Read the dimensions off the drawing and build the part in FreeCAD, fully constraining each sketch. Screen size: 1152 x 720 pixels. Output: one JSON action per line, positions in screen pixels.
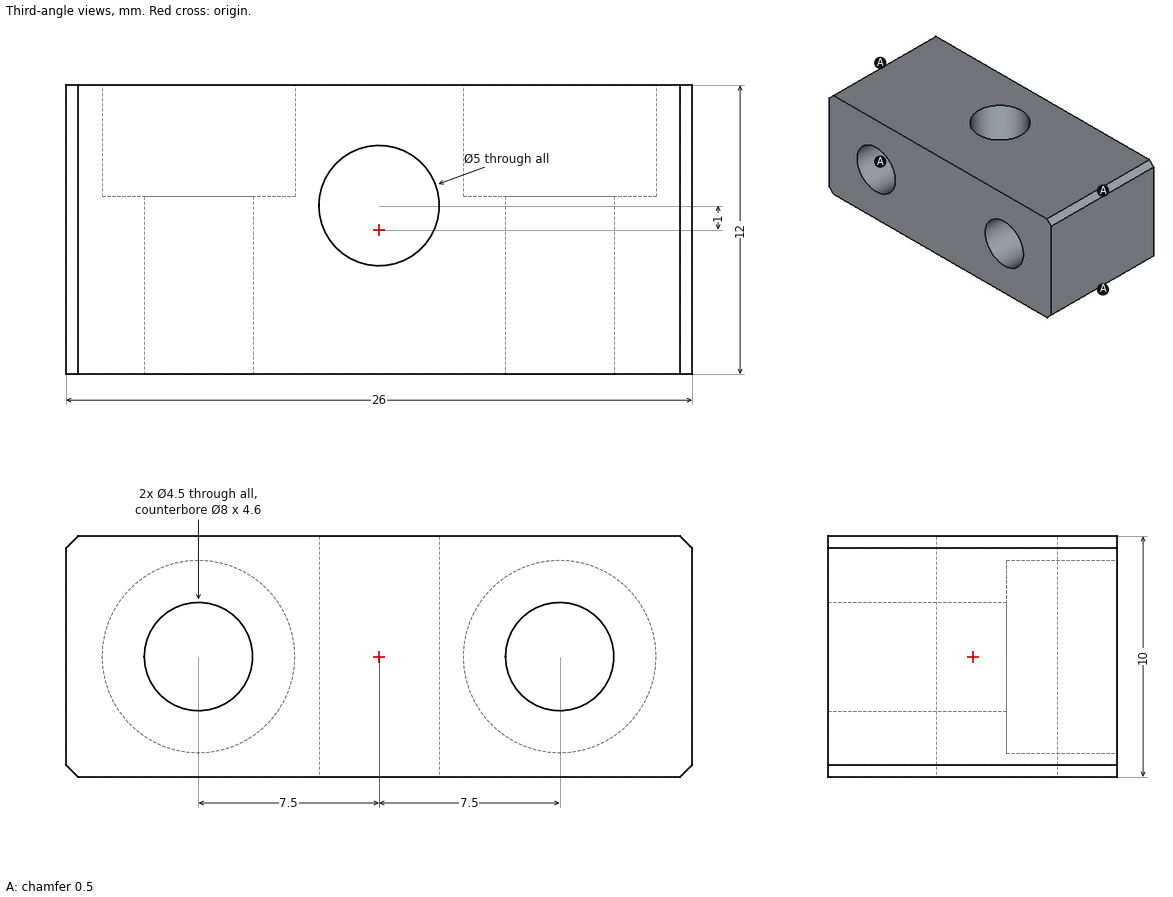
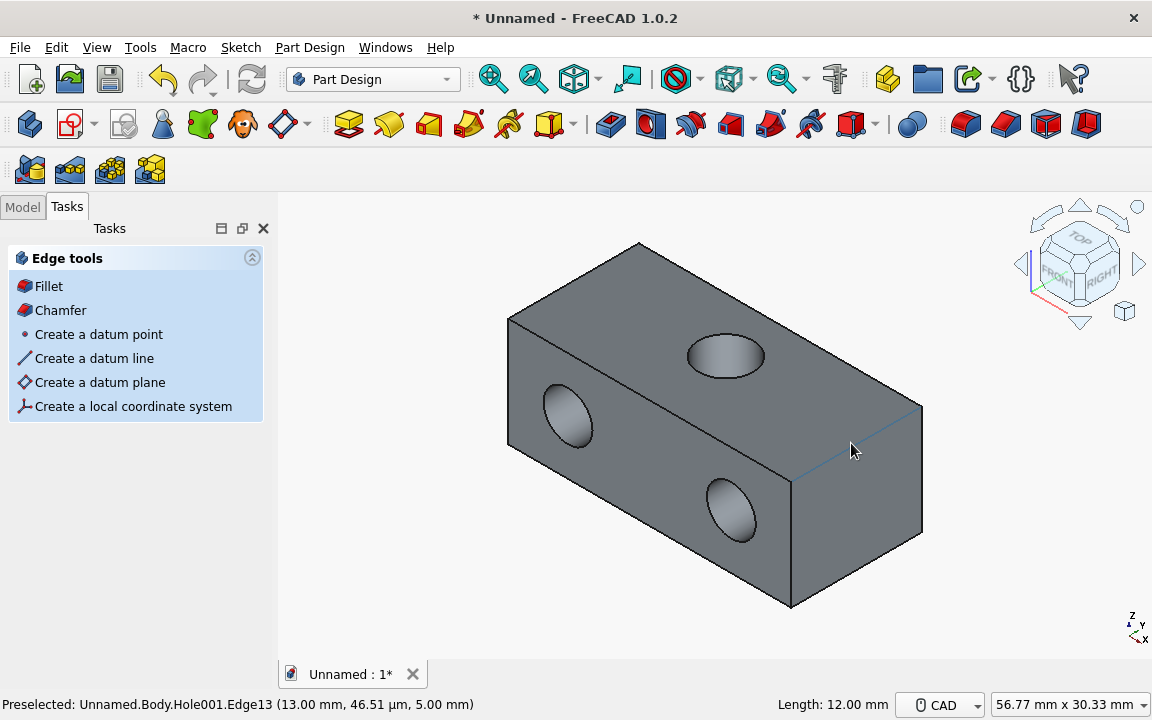
{"action": "key", "text": "2"}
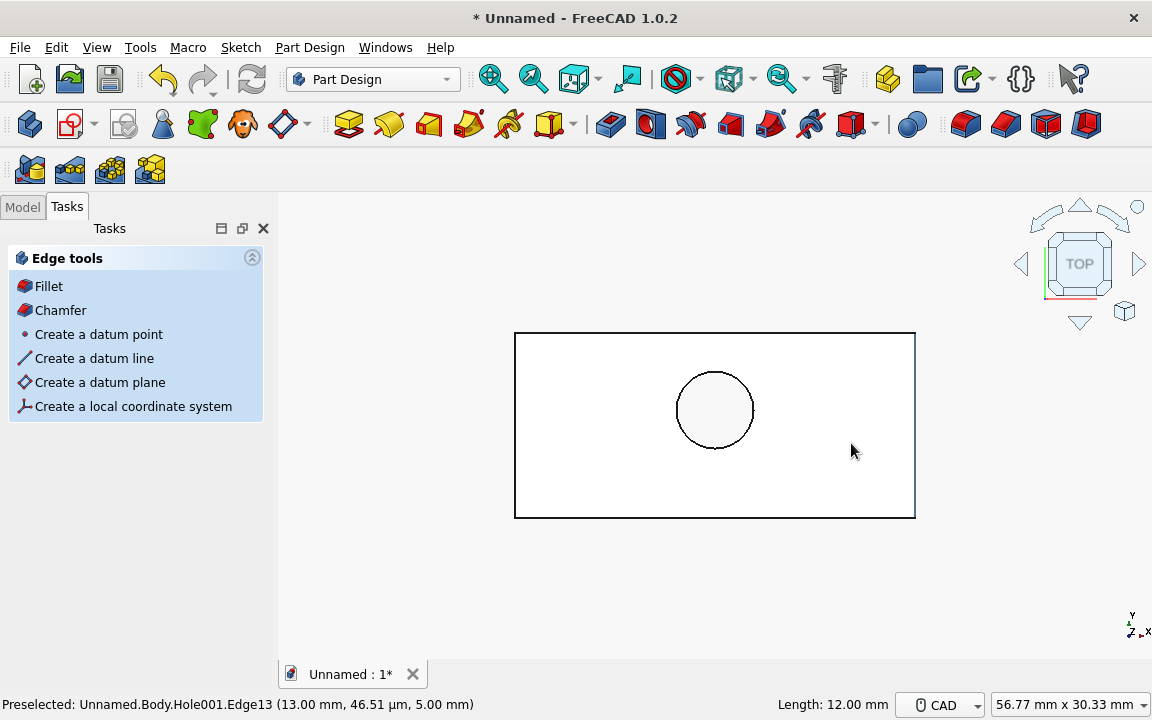
{"action": "left_click", "coordinate": [515, 424], "text": "ctrl"}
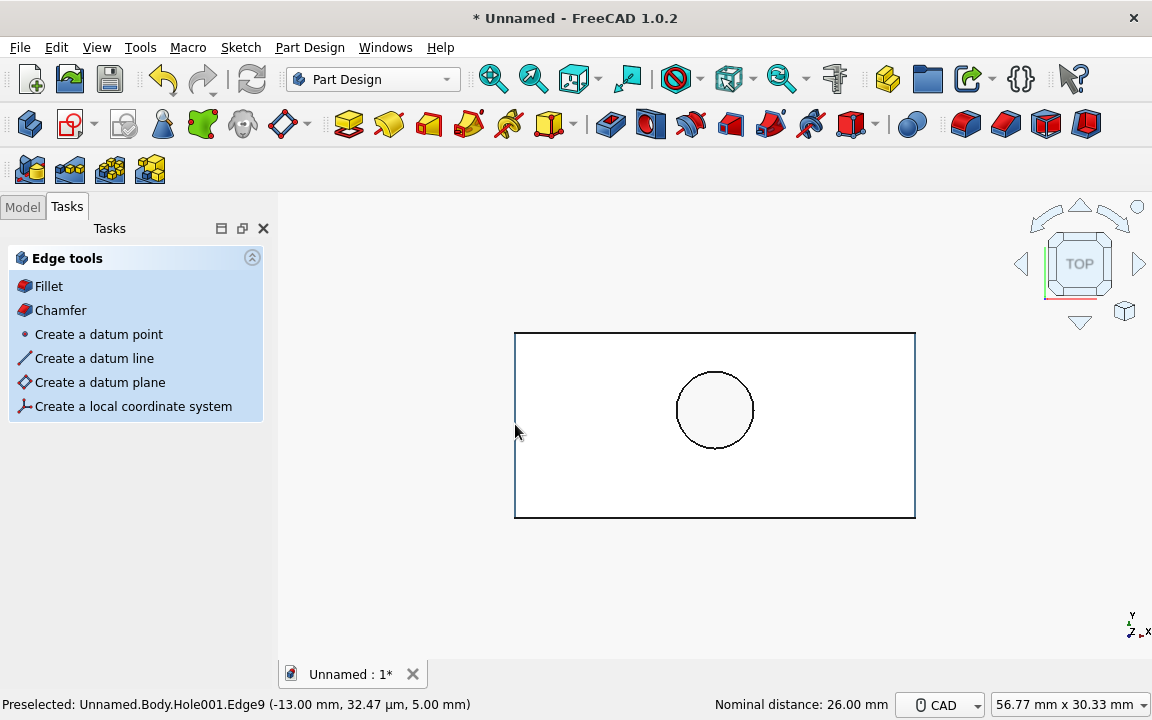
{"action": "key", "text": "0"}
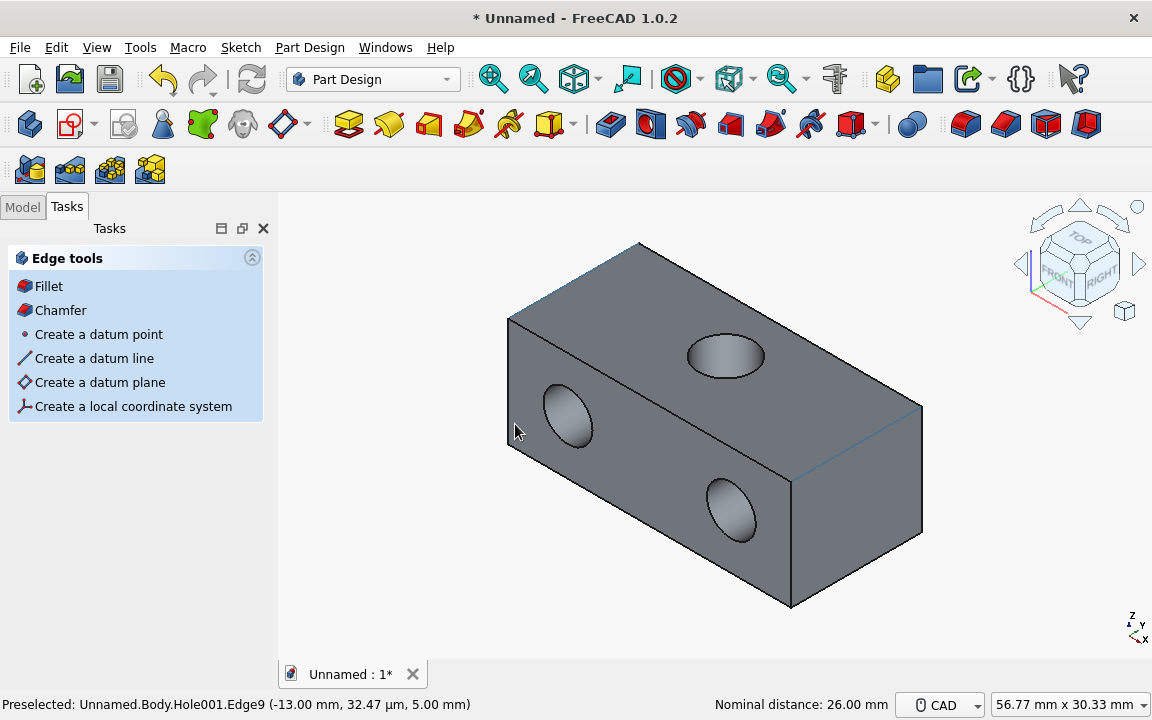
{"action": "key", "text": "1"}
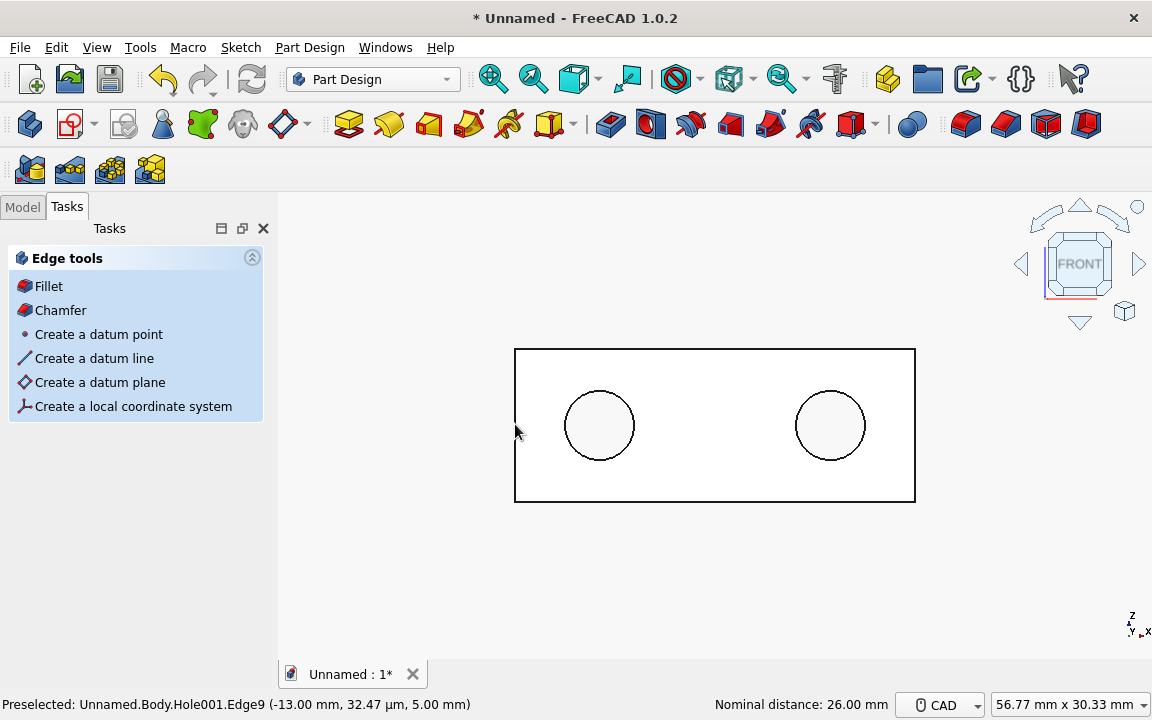
{"action": "key", "text": "3"}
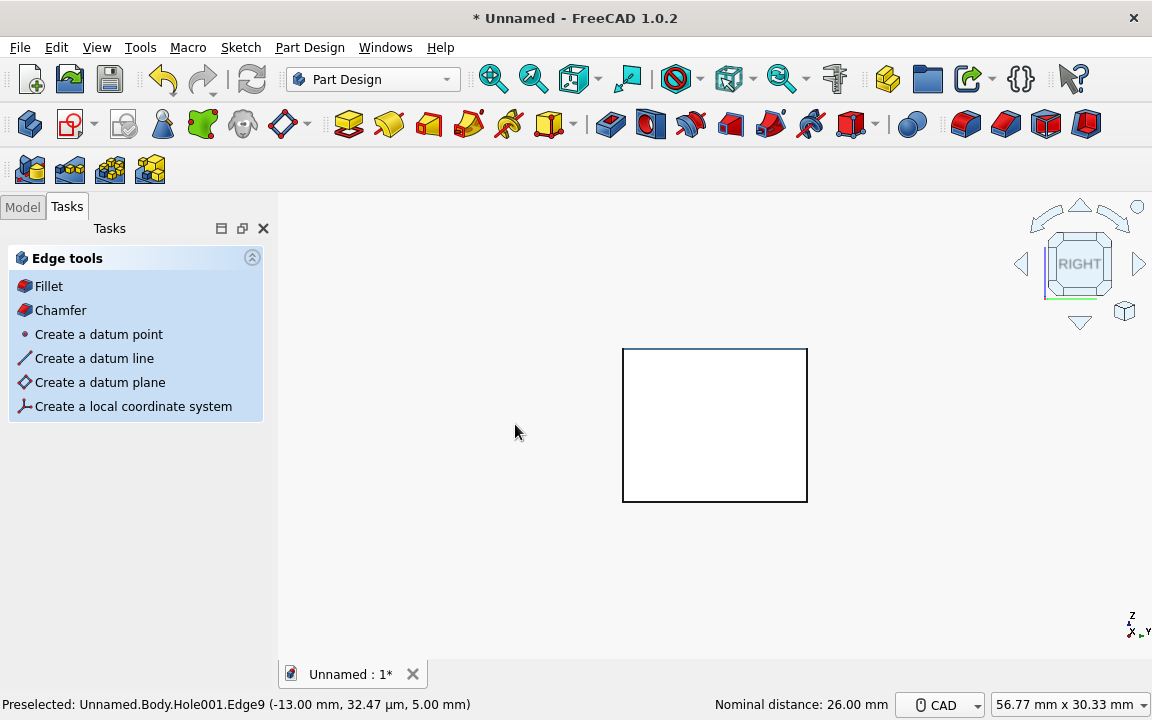
{"action": "key", "text": "v f"}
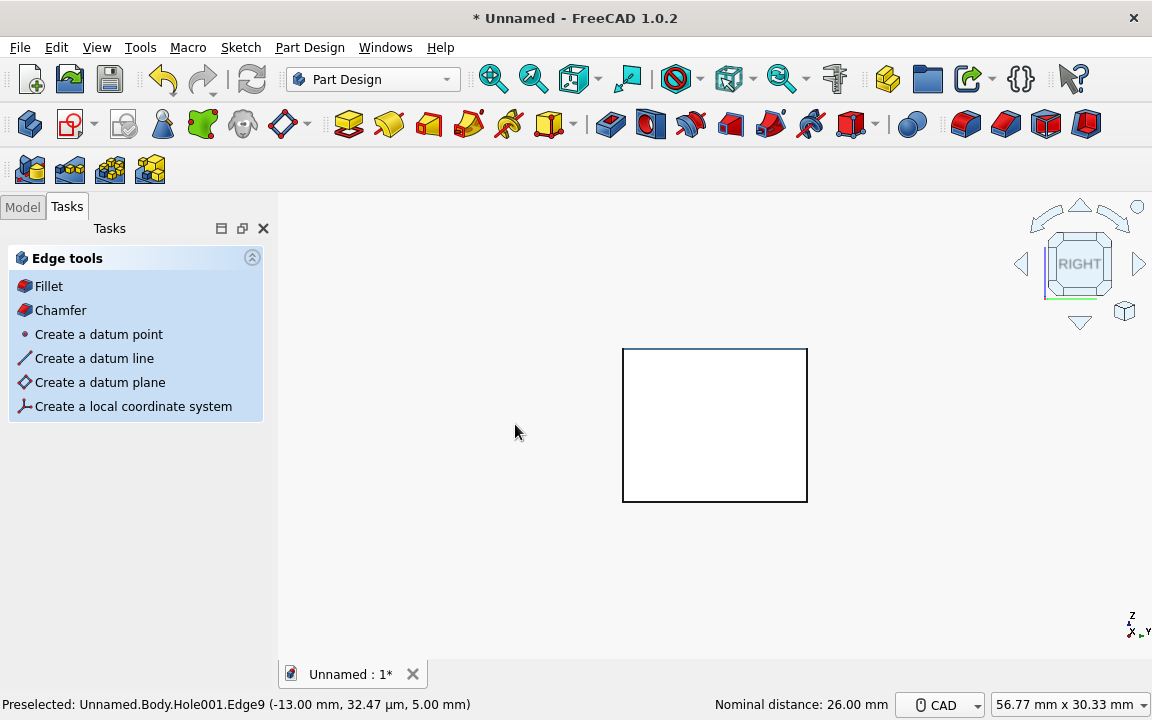
{"action": "left_click", "coordinate": [715, 501], "text": "ctrl"}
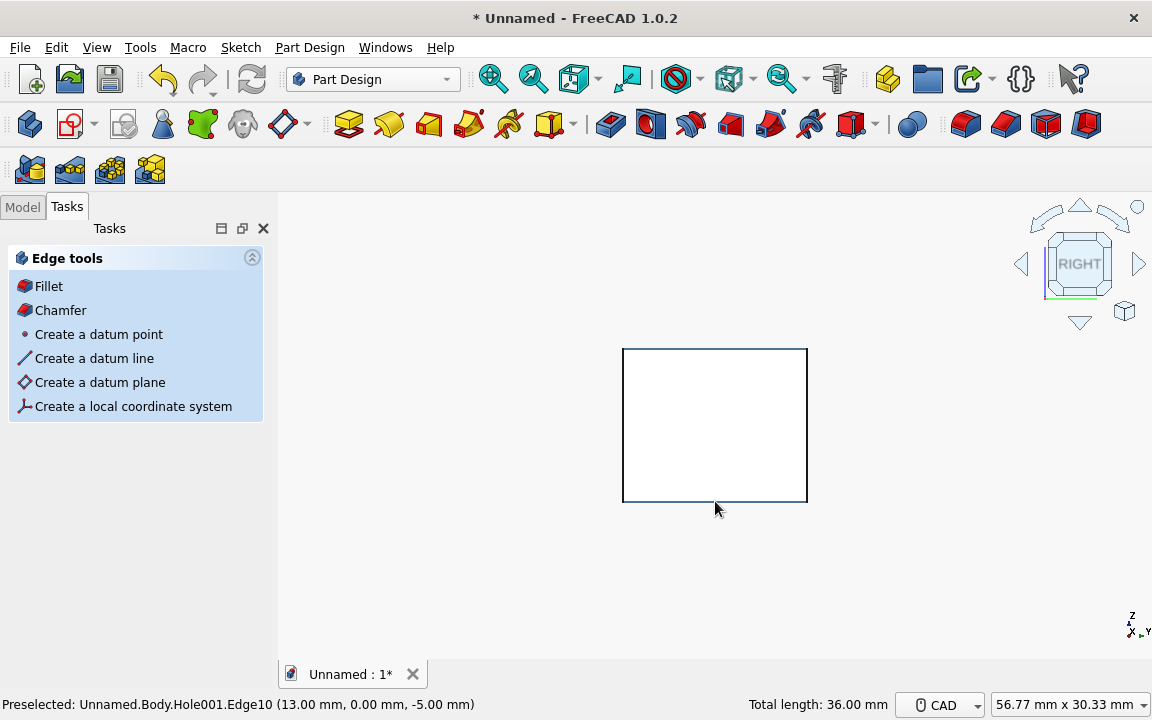
{"action": "key", "text": "5"}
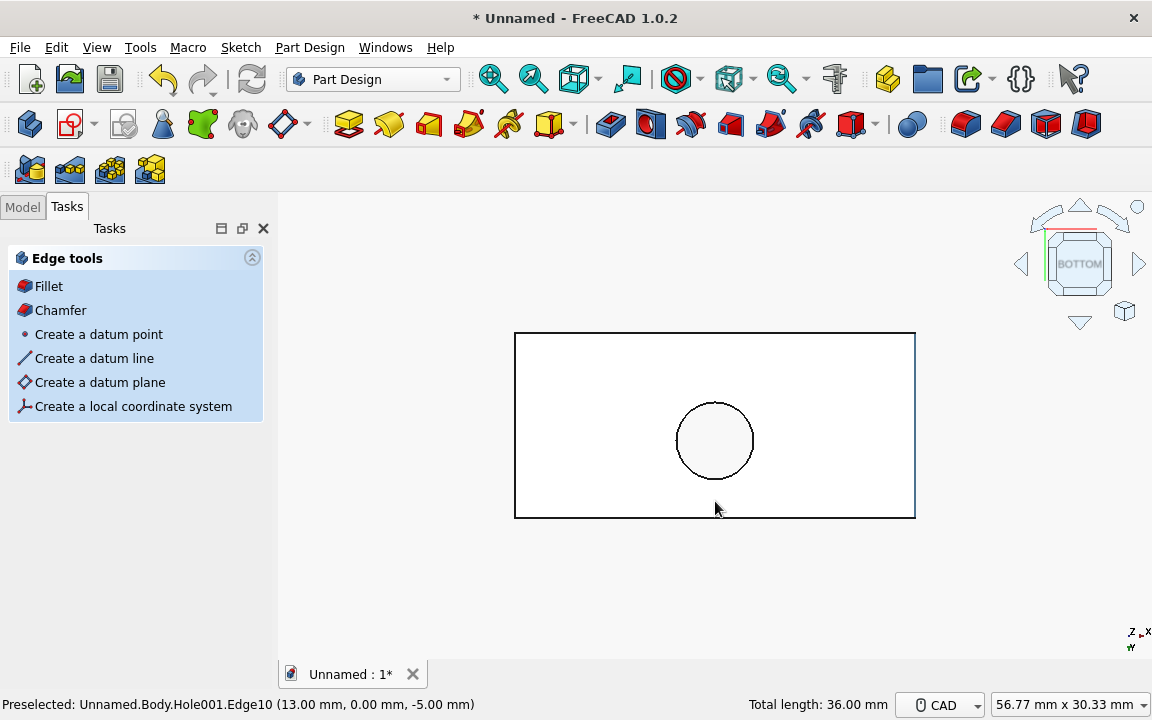
{"action": "left_click", "coordinate": [515, 424], "text": "ctrl"}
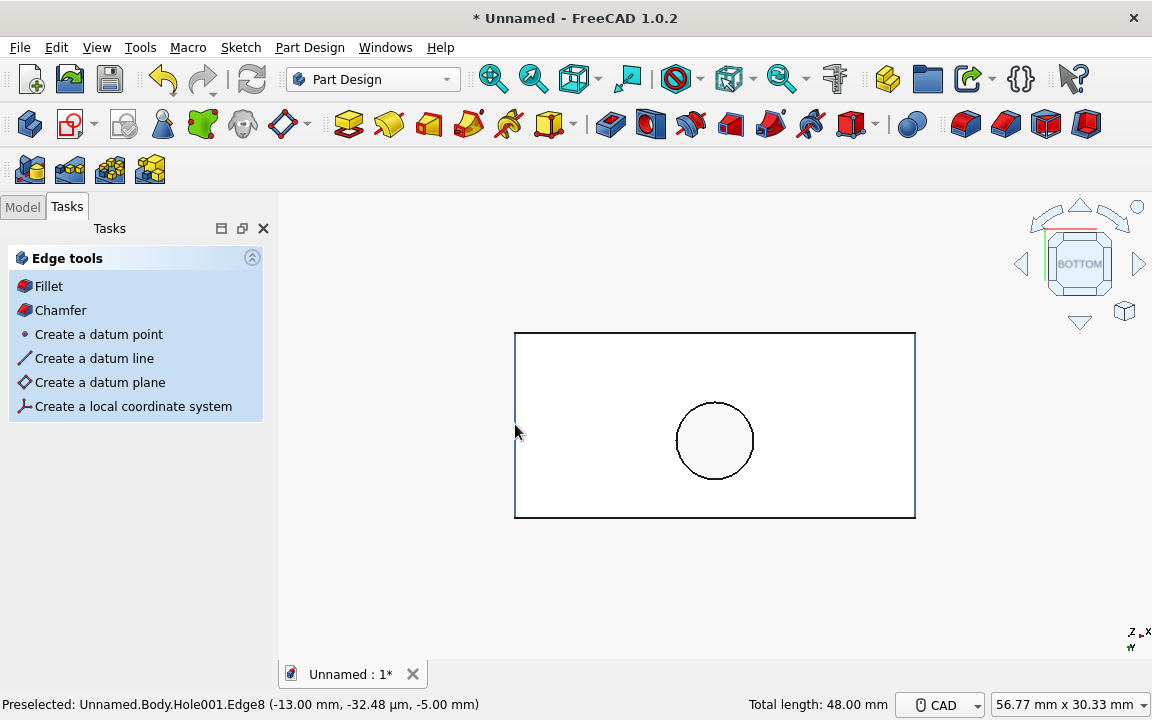
{"action": "left_click", "coordinate": [1006, 124]}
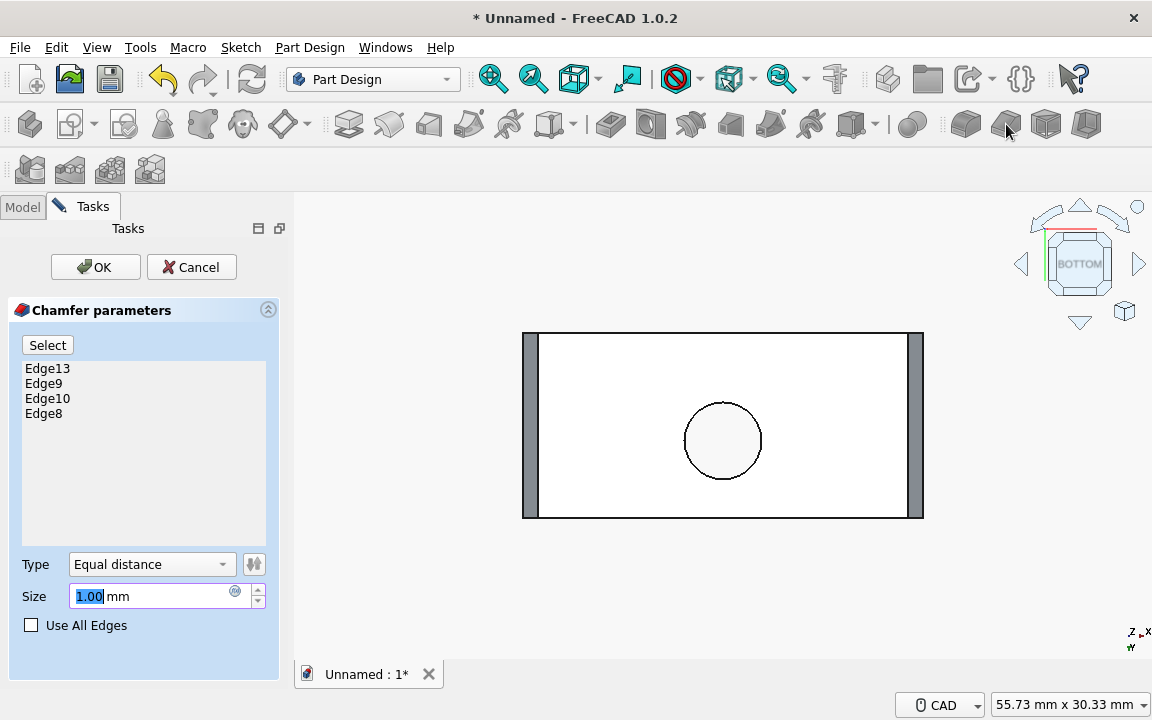
{"action": "type", "text": "0.5"}
{"action": "key", "text": "Tab"}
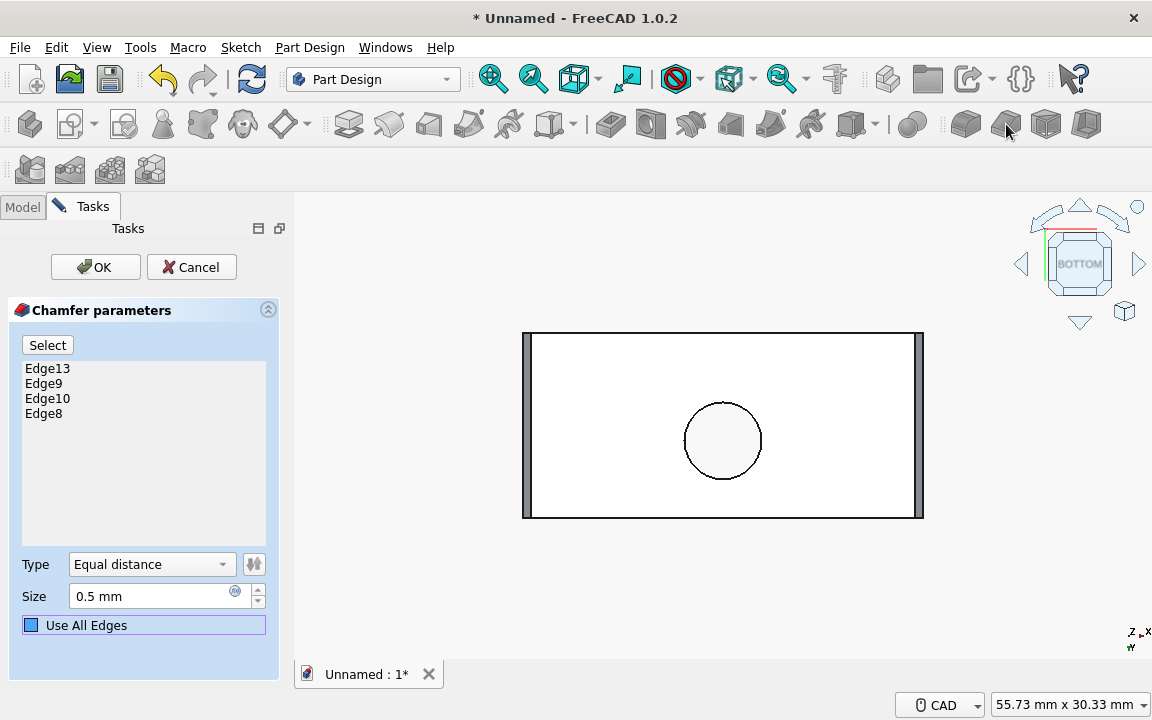
{"action": "left_click", "coordinate": [96, 267]}